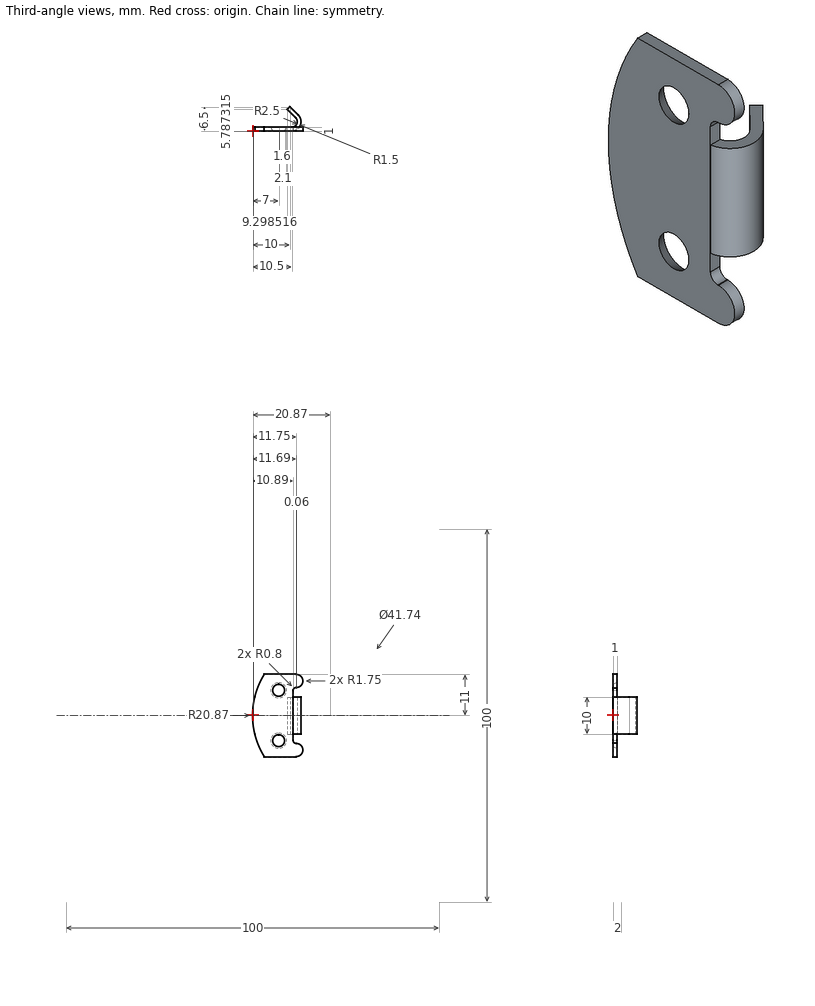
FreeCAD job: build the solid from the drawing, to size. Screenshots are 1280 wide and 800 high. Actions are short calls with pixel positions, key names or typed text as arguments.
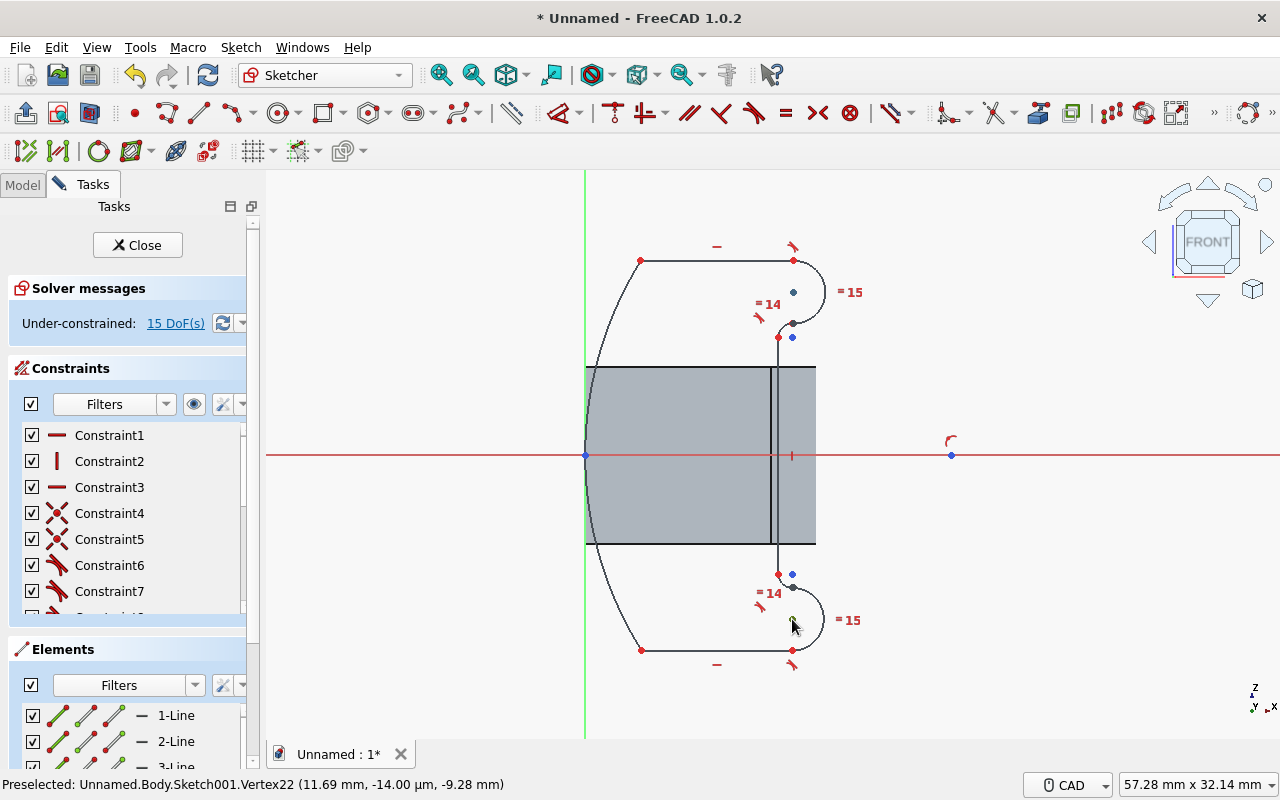
click(353, 455)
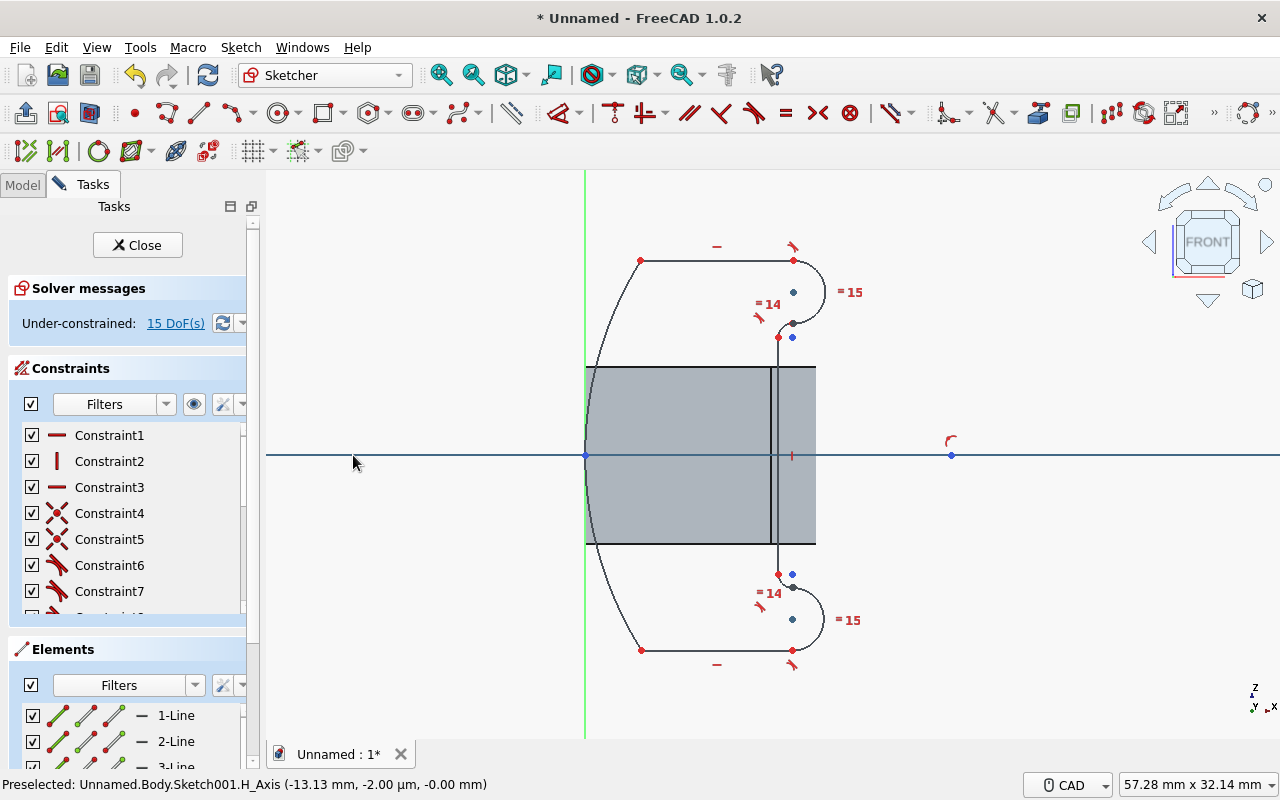
click(818, 114)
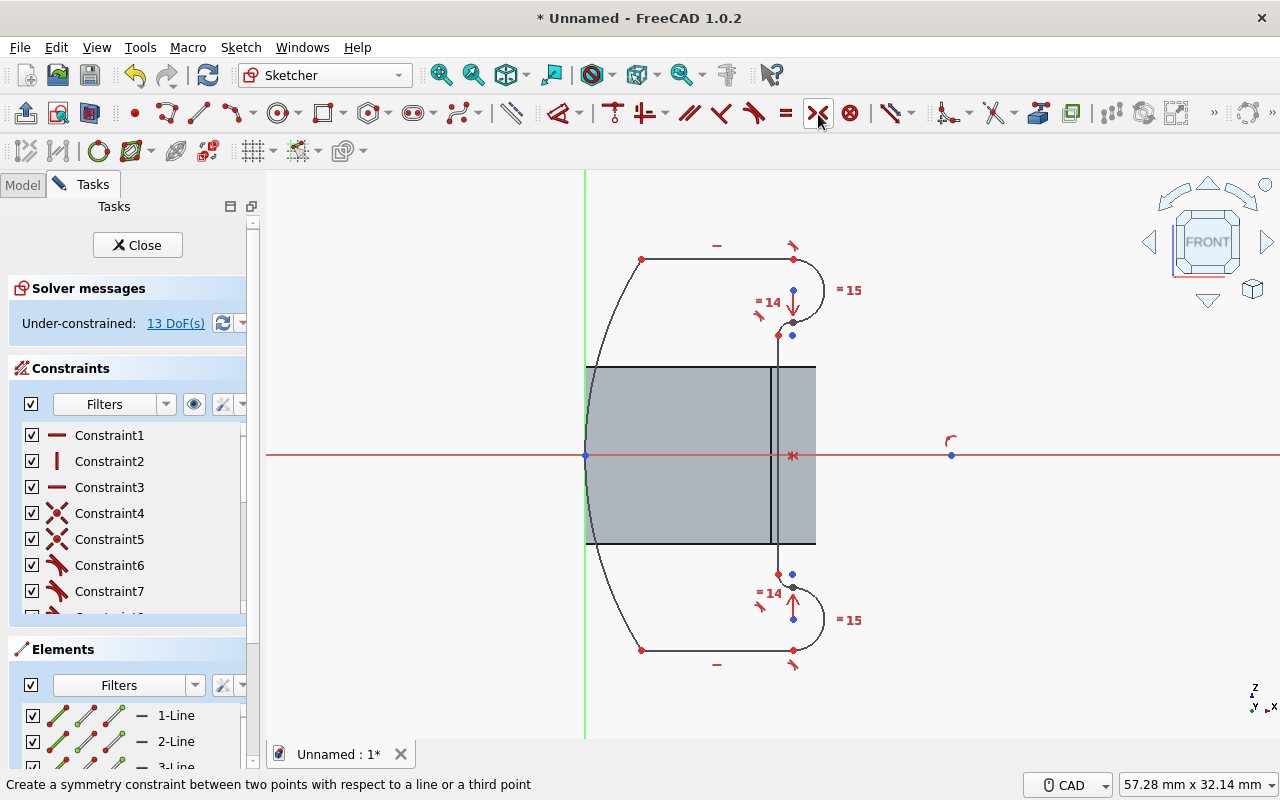
click(558, 114)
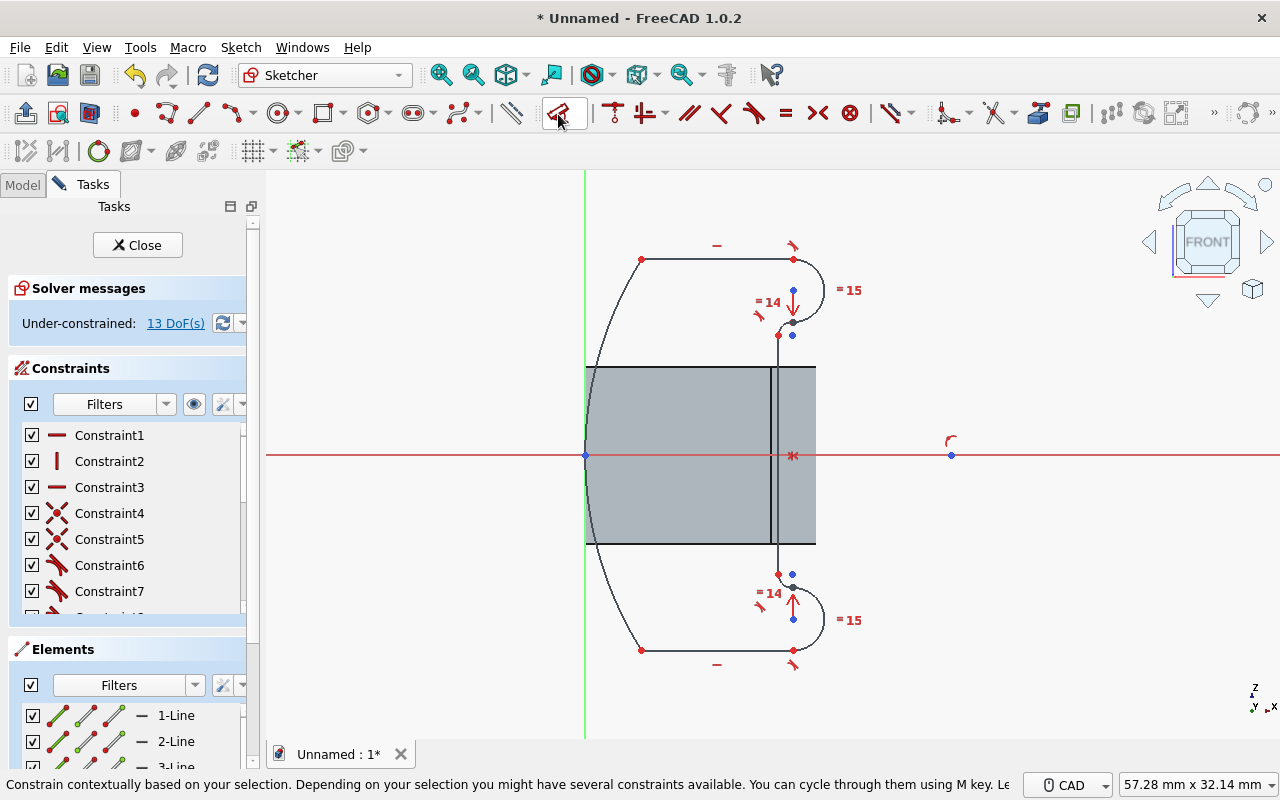
scroll(819, 309, up, 2)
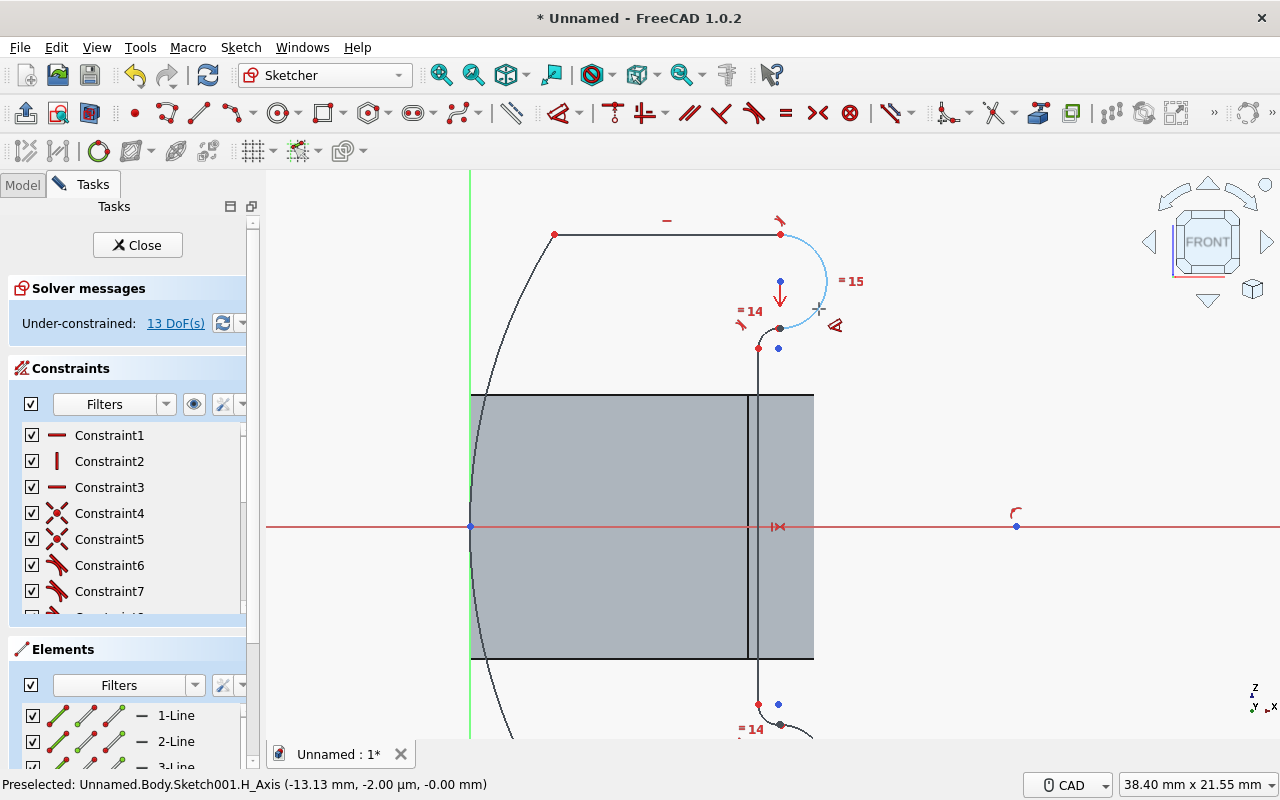
click(818, 309)
click(844, 328)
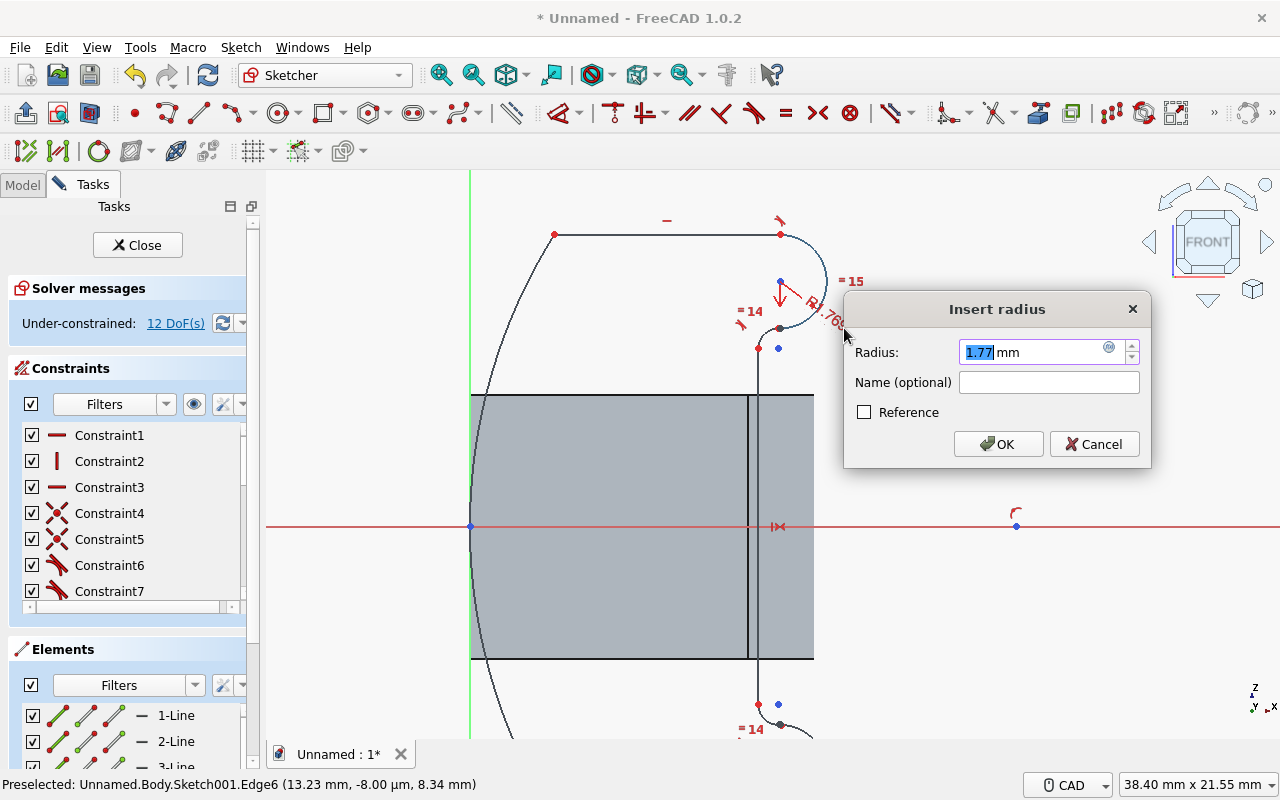
text(1.75)
key(Return)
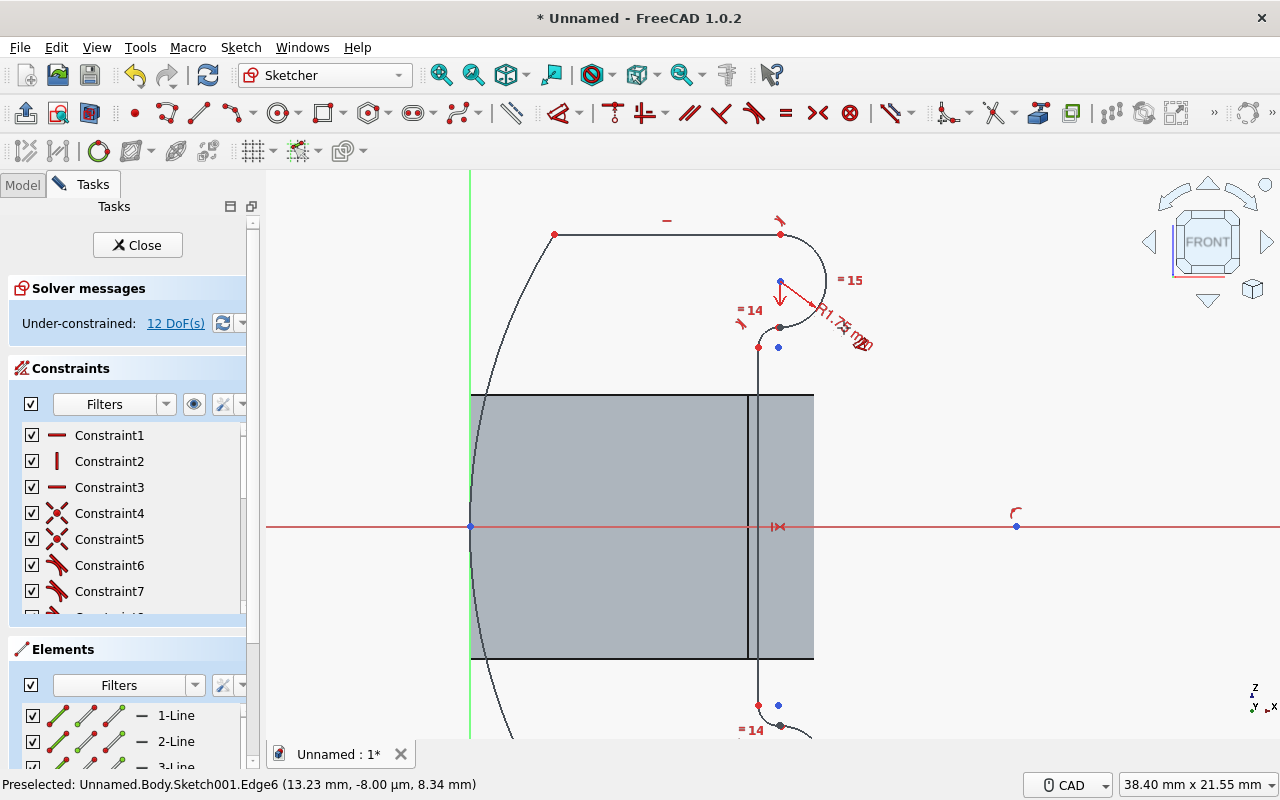
scroll(770, 330, up, 4)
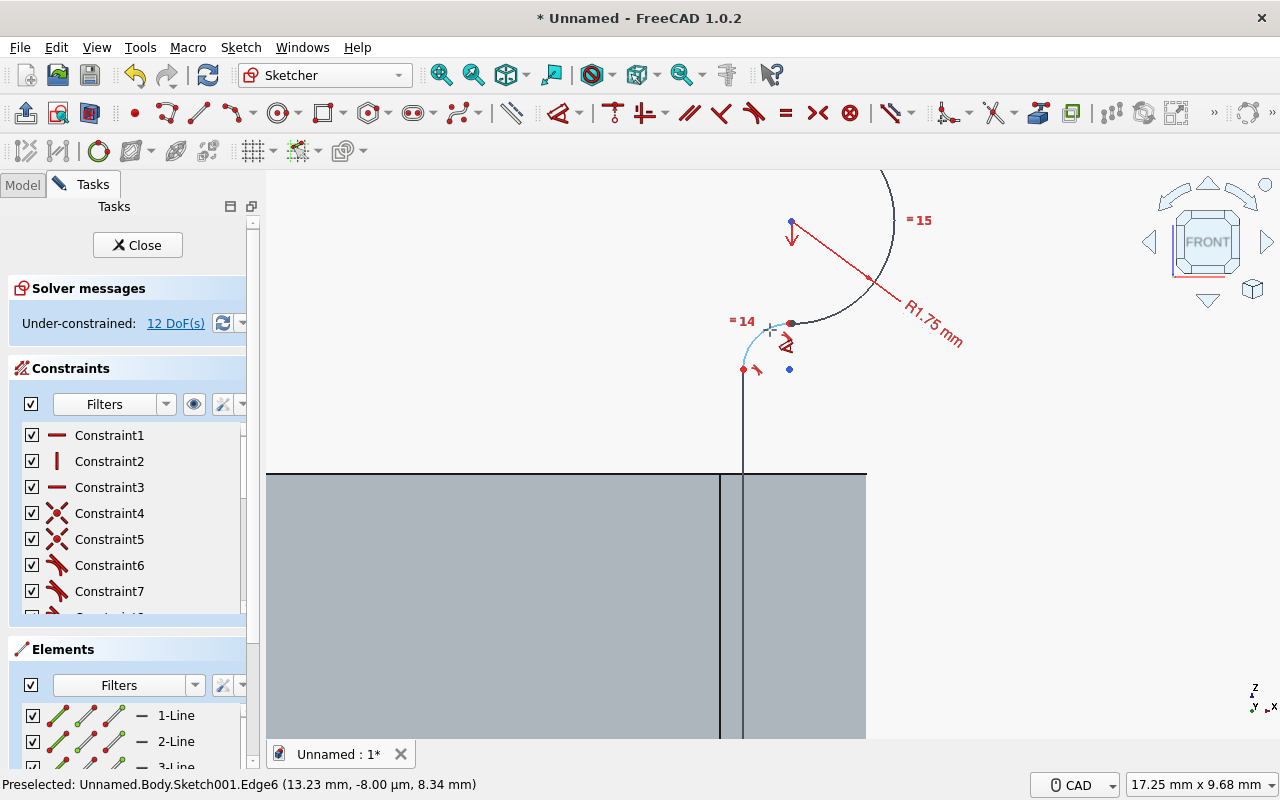
click(768, 329)
click(753, 301)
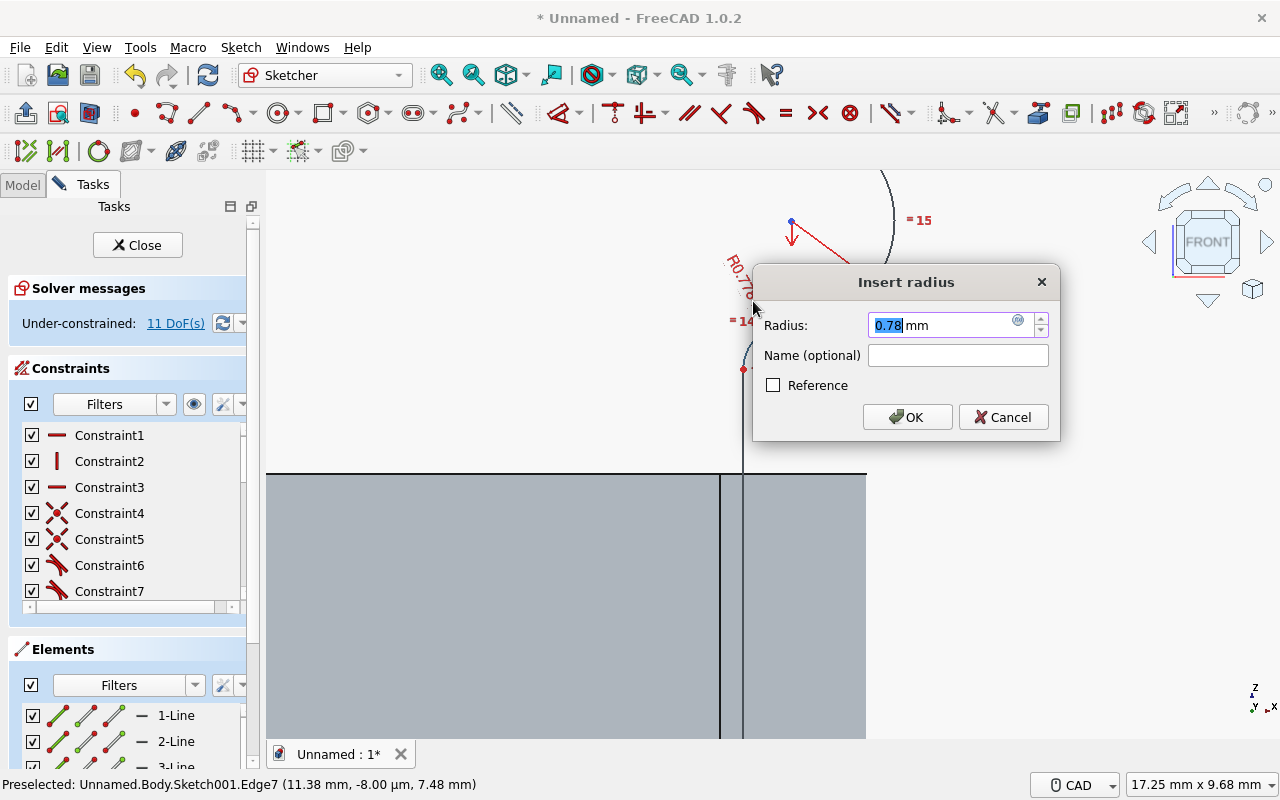
text(0.8)
key(Return)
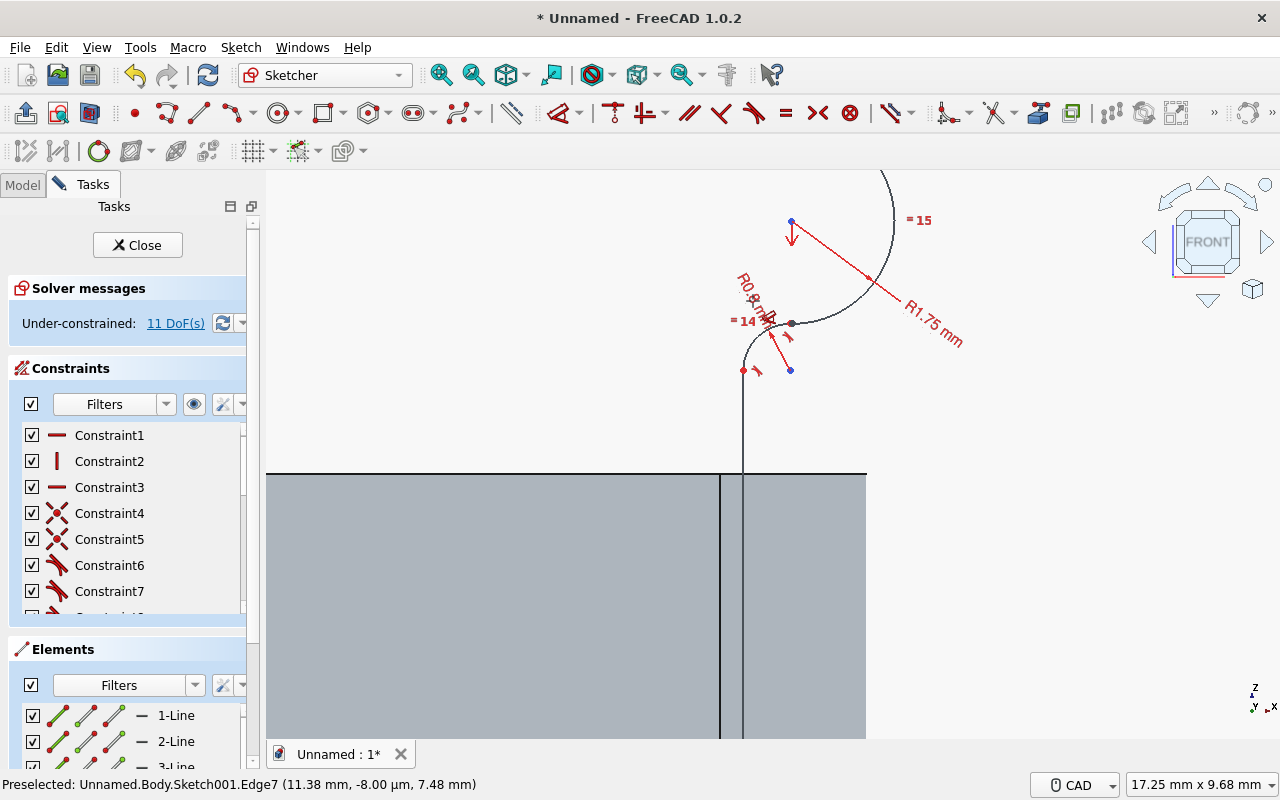
scroll(793, 320, down, 6)